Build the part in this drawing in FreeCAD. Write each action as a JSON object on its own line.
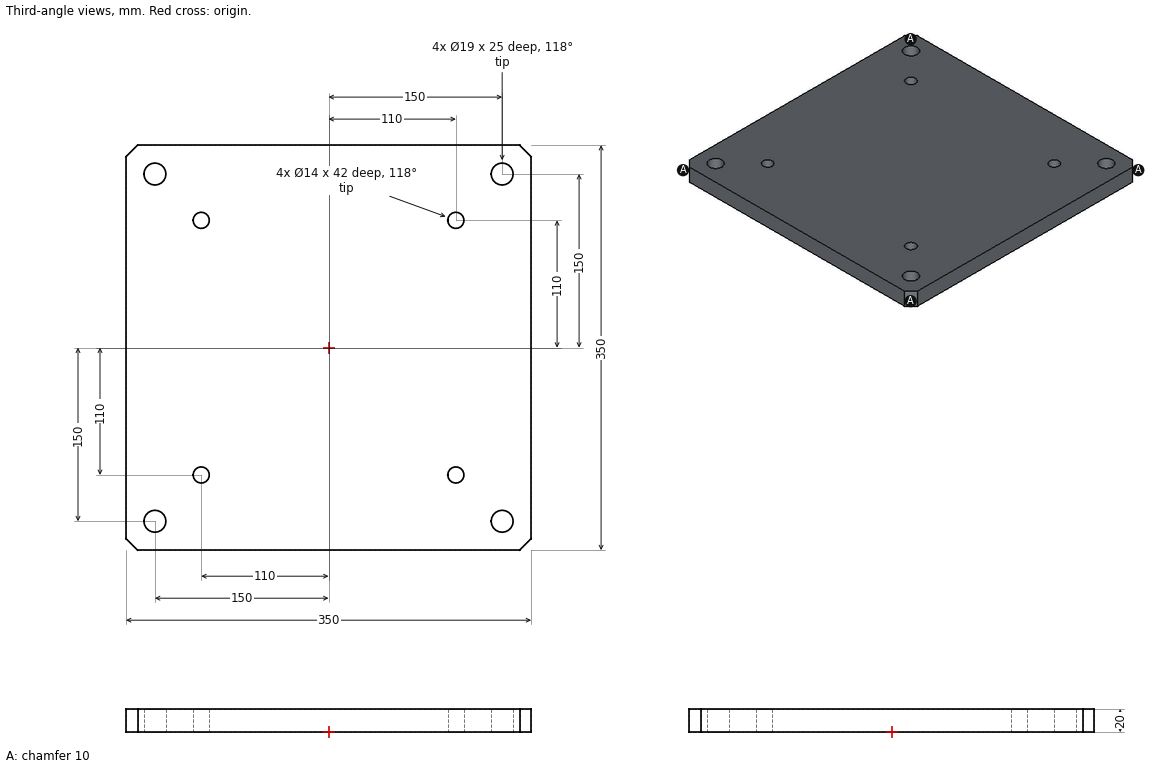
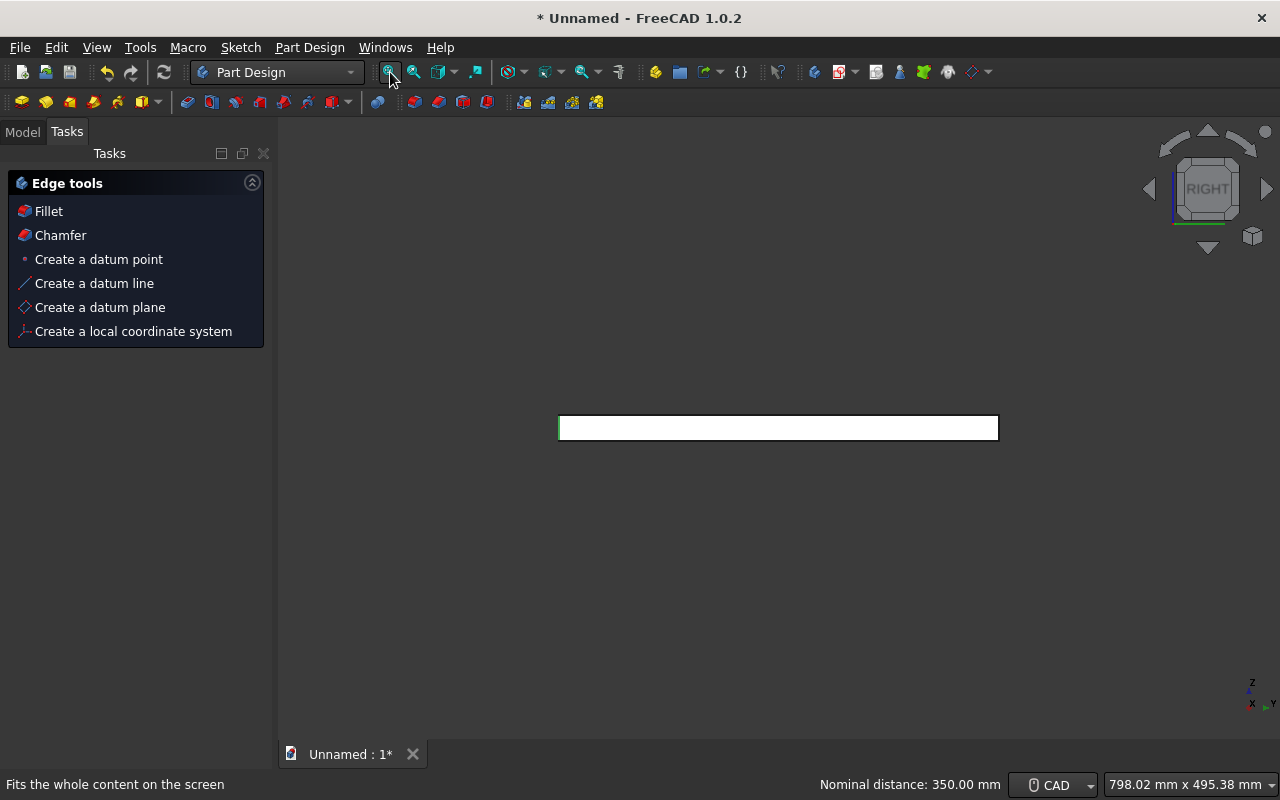
{"action": "left_click", "coordinate": [999, 427], "text": "ctrl"}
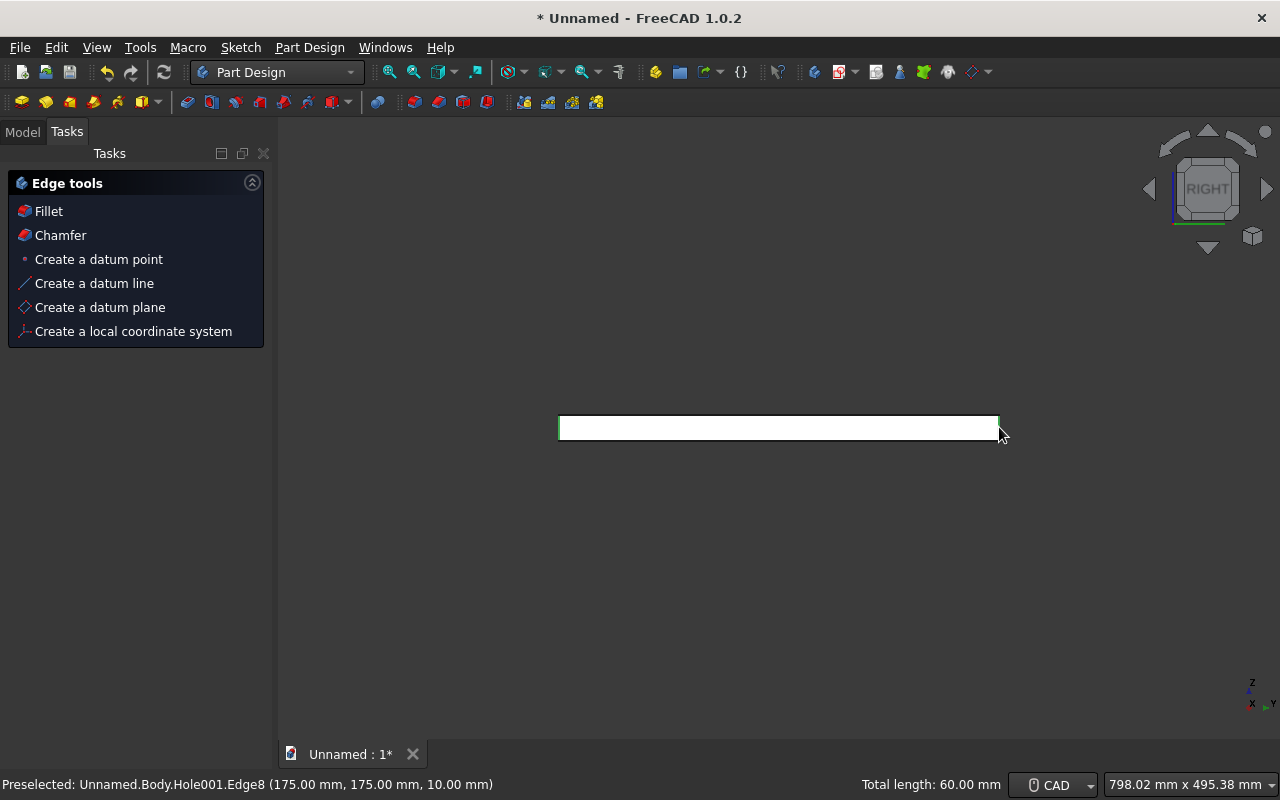
{"action": "key", "text": "5"}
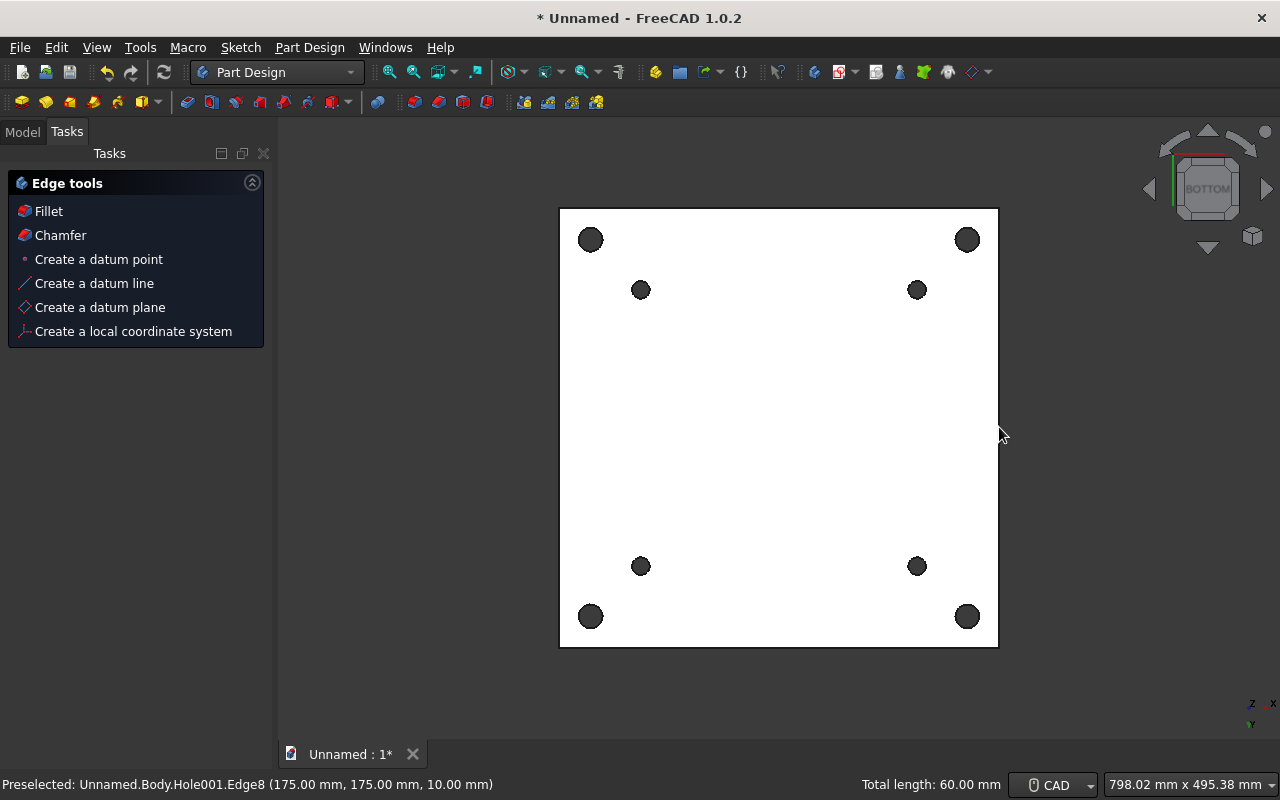
{"action": "key", "text": "4"}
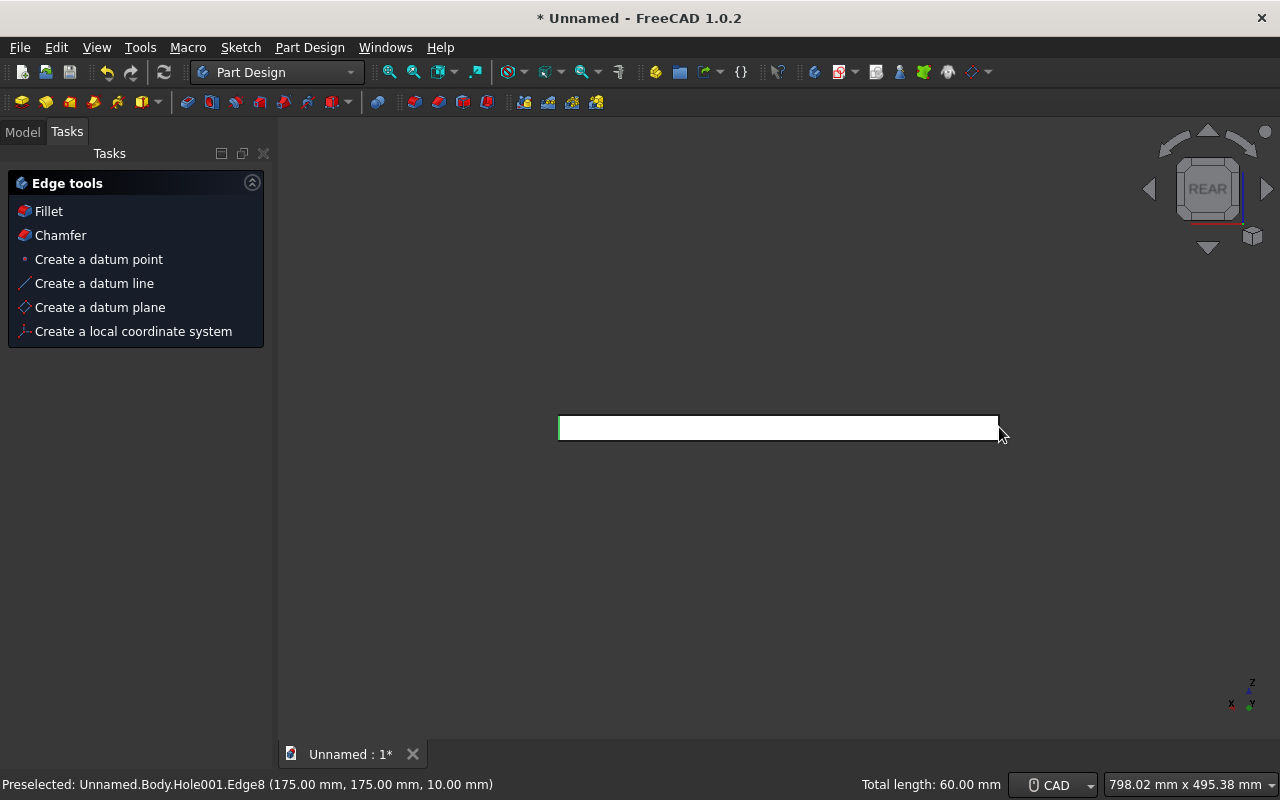
{"action": "left_click", "coordinate": [390, 72]}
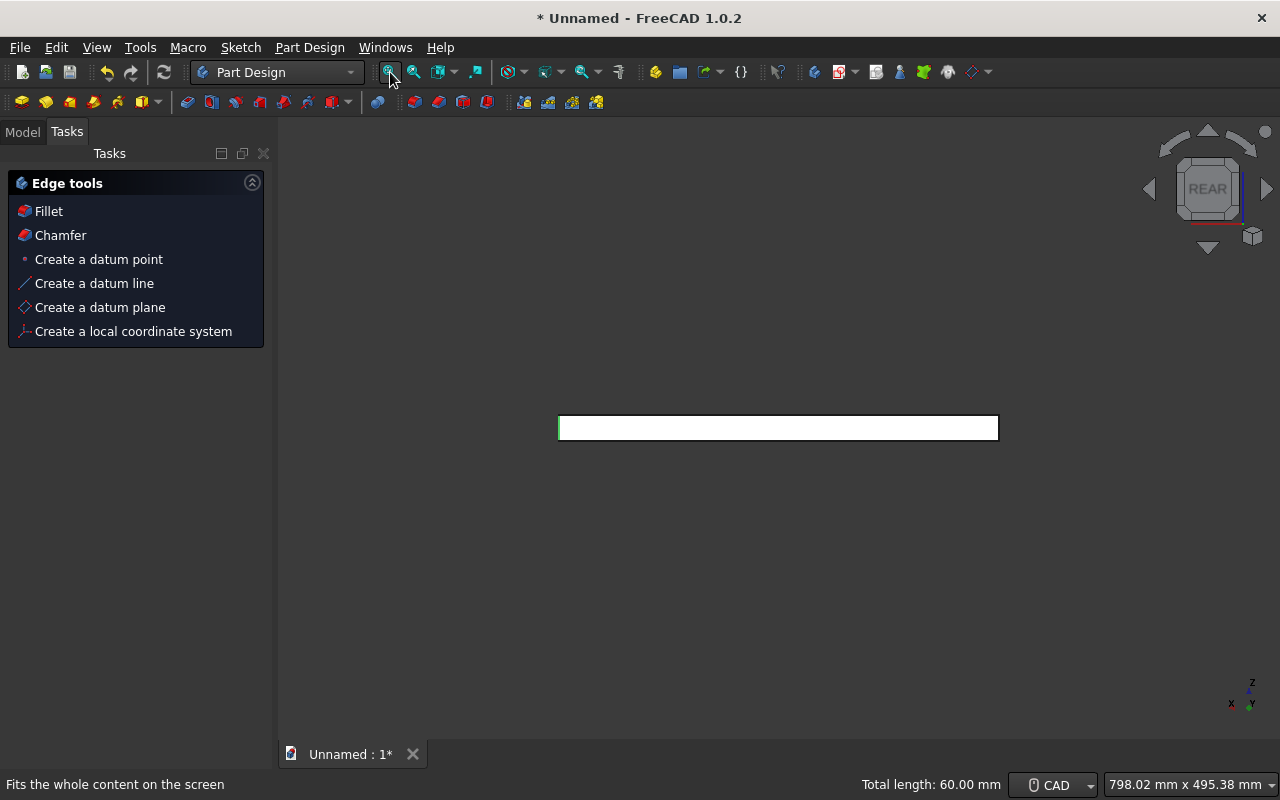
{"action": "left_click", "coordinate": [999, 427], "text": "ctrl"}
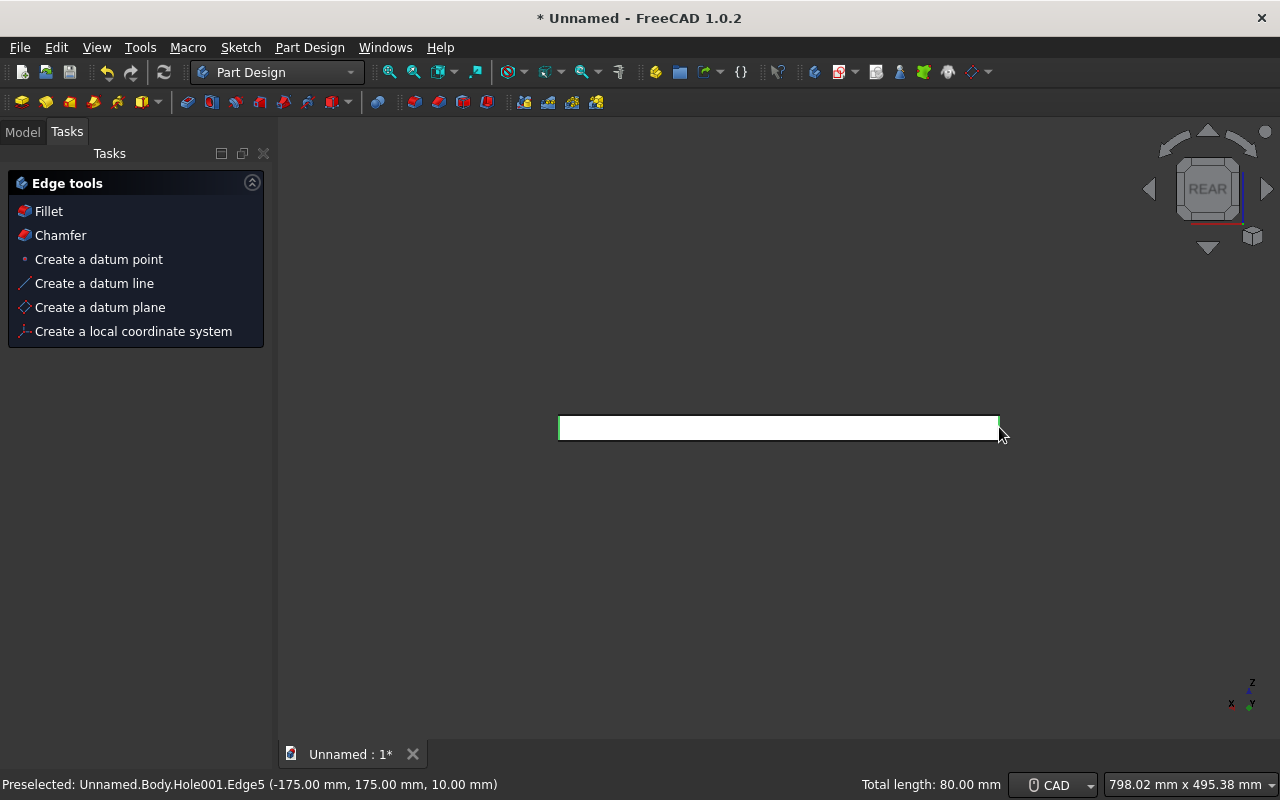
{"action": "left_click", "coordinate": [440, 102]}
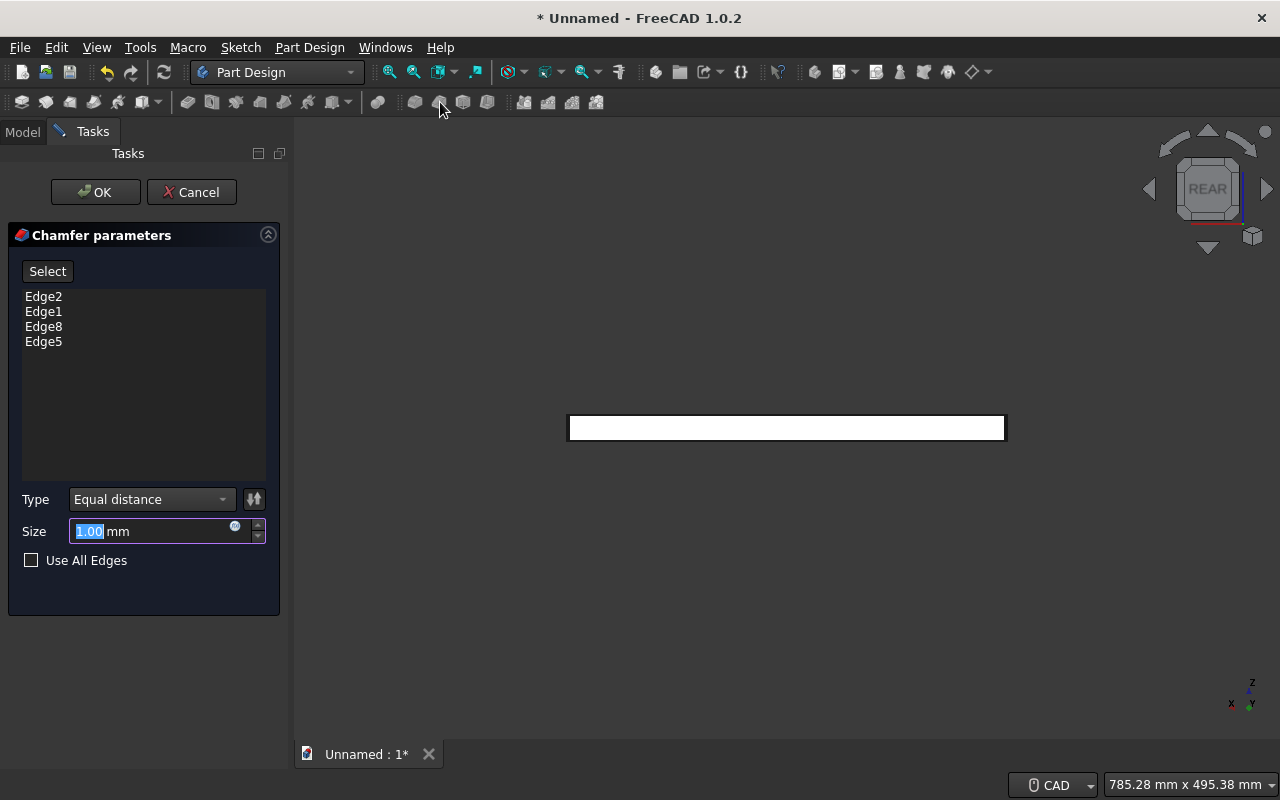
{"action": "type", "text": "10"}
{"action": "key", "text": "Tab"}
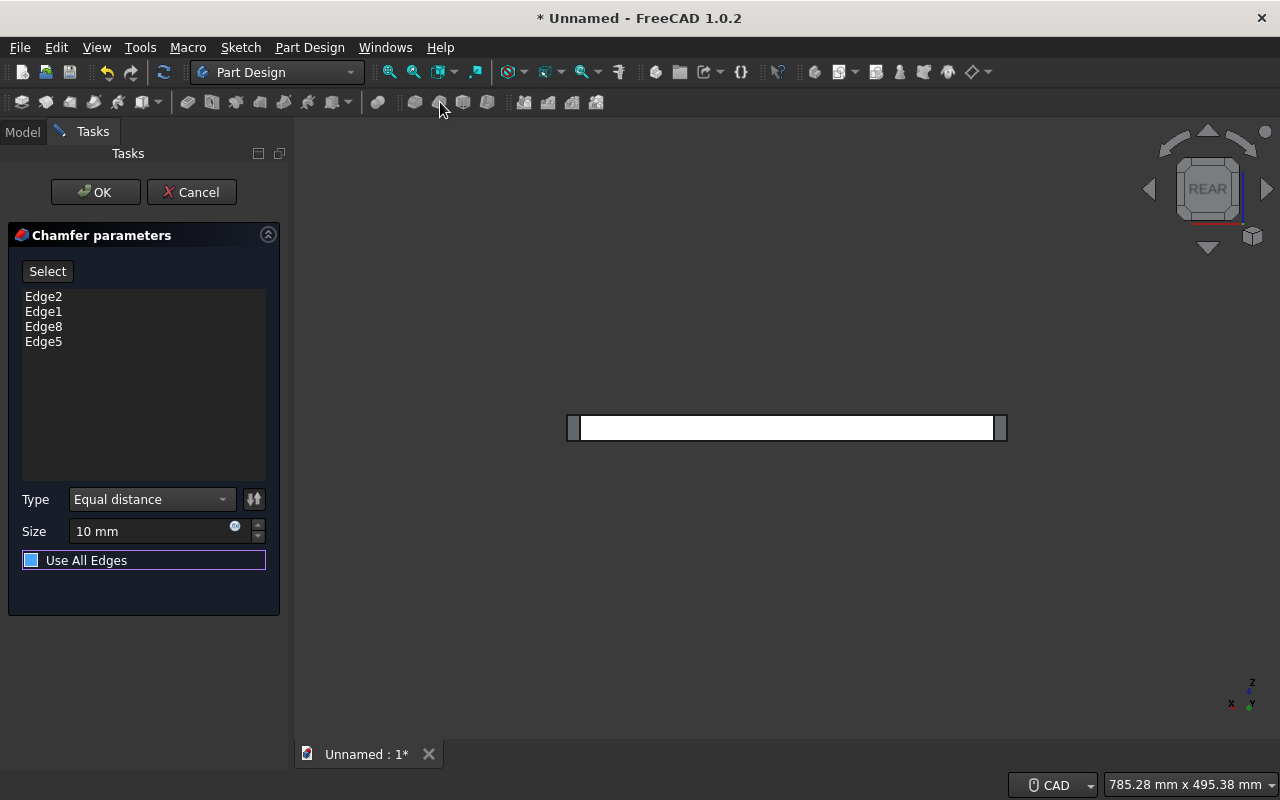
{"action": "left_click", "coordinate": [96, 192]}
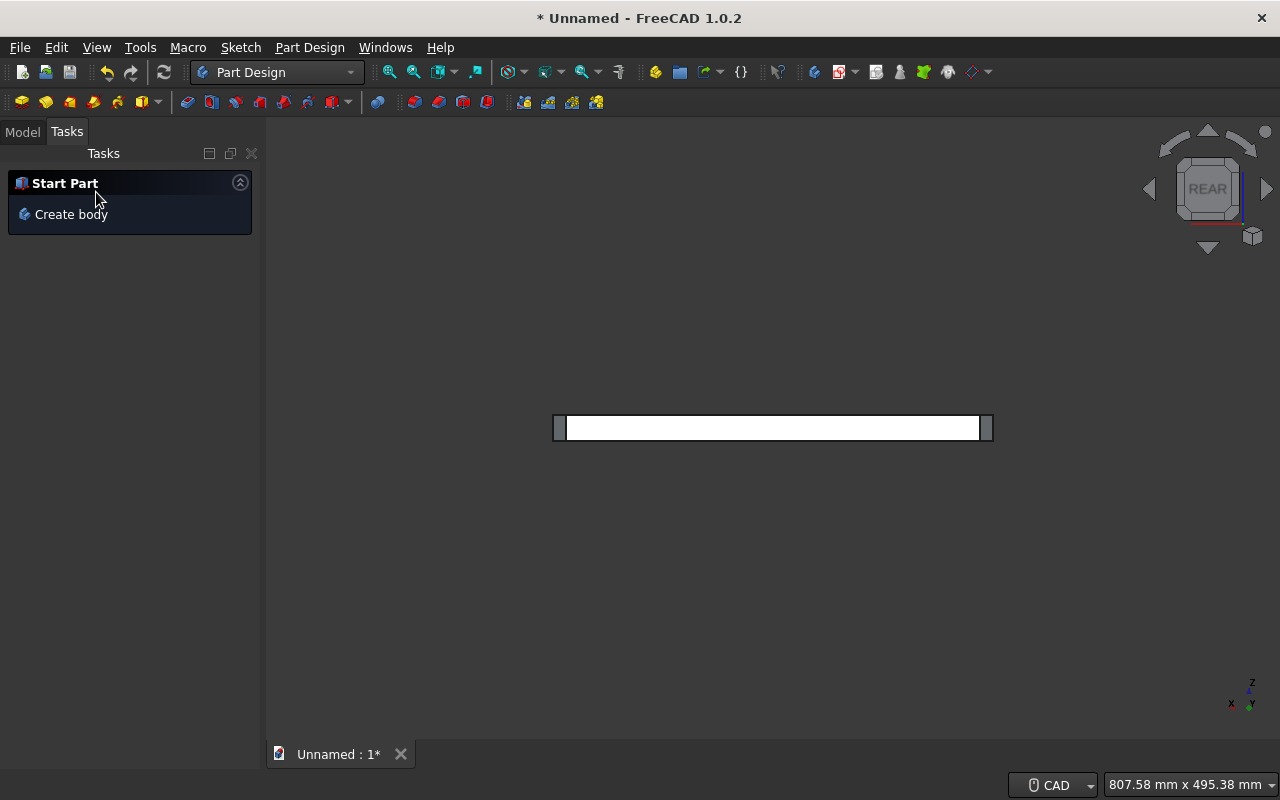
{"action": "key", "text": "0"}